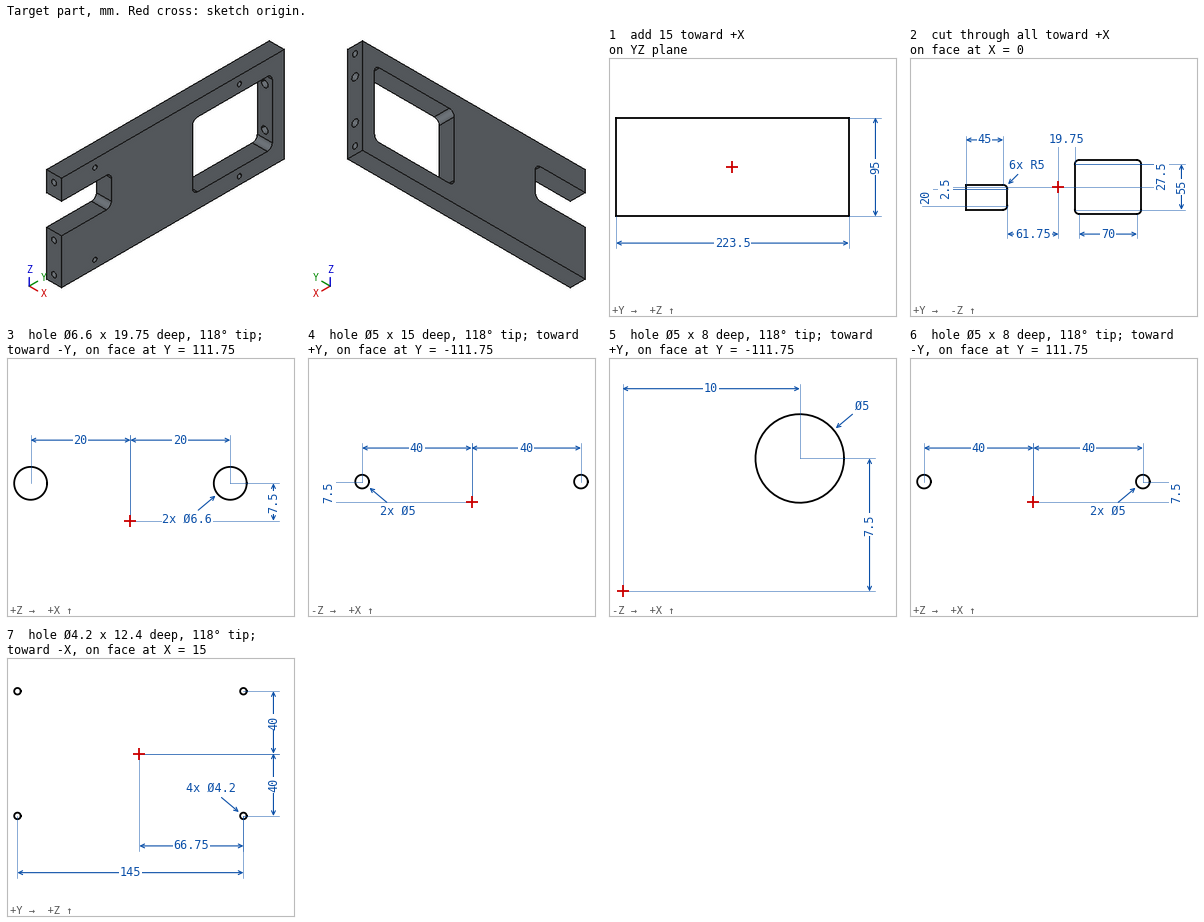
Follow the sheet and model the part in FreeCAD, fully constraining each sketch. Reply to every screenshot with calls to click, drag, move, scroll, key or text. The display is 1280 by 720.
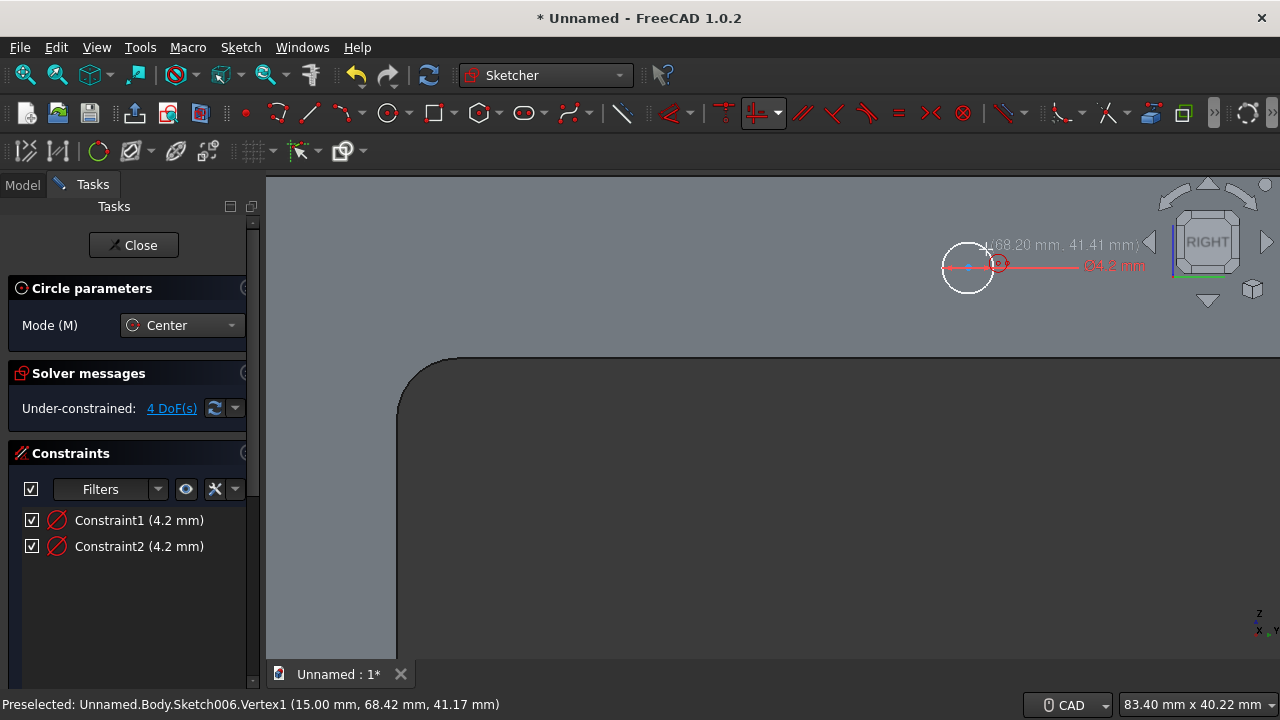
scroll(971, 268, down, 6)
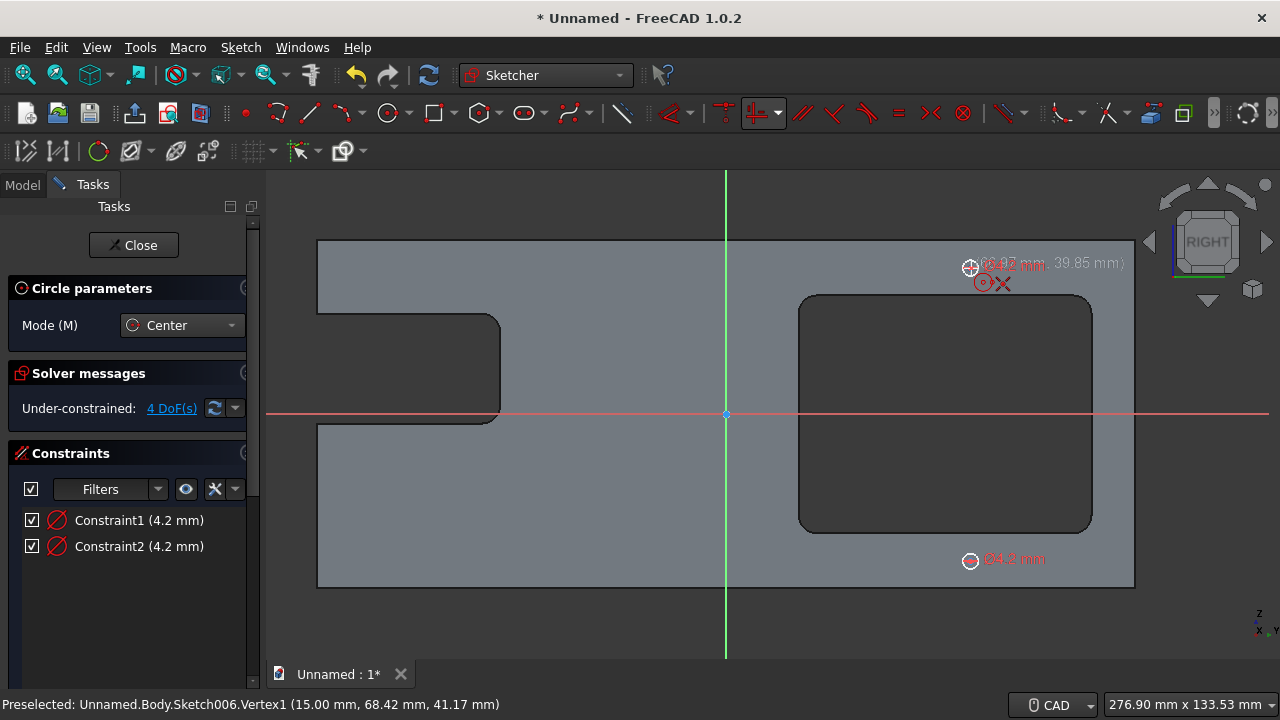
scroll(440, 561, up, 6)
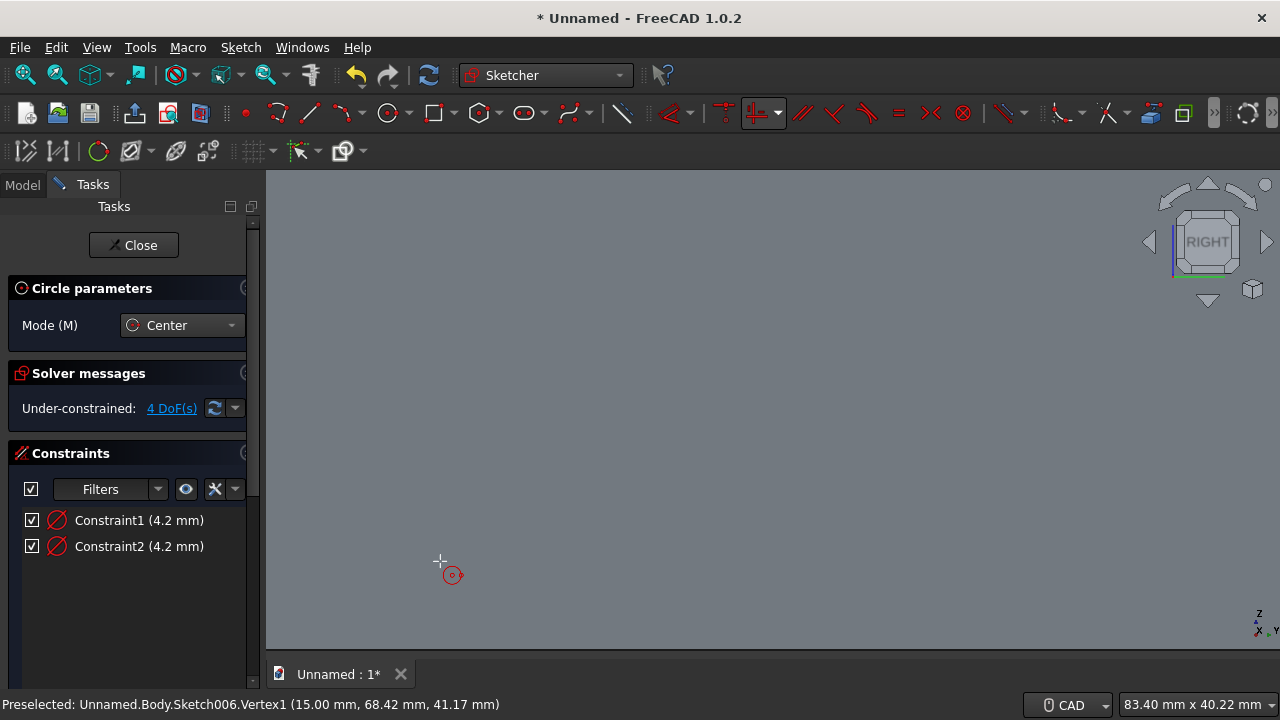
click(439, 559)
move(457, 541)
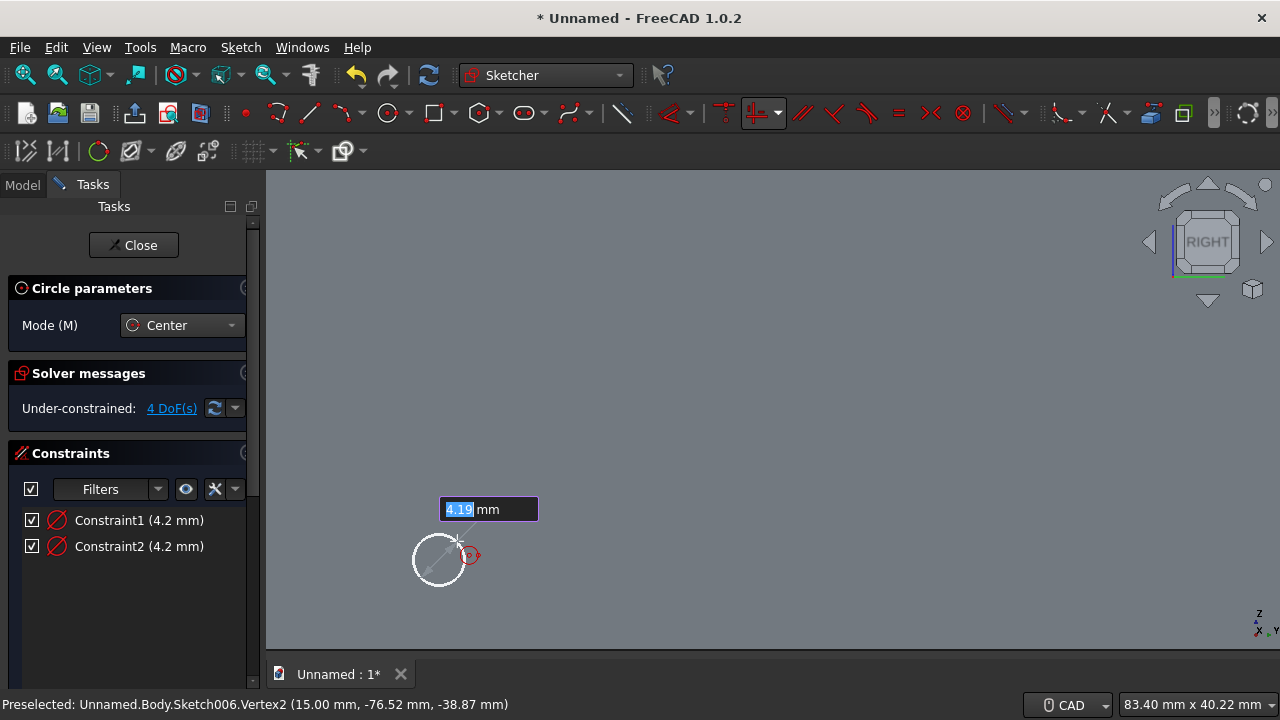
text(4.2)
key(Return)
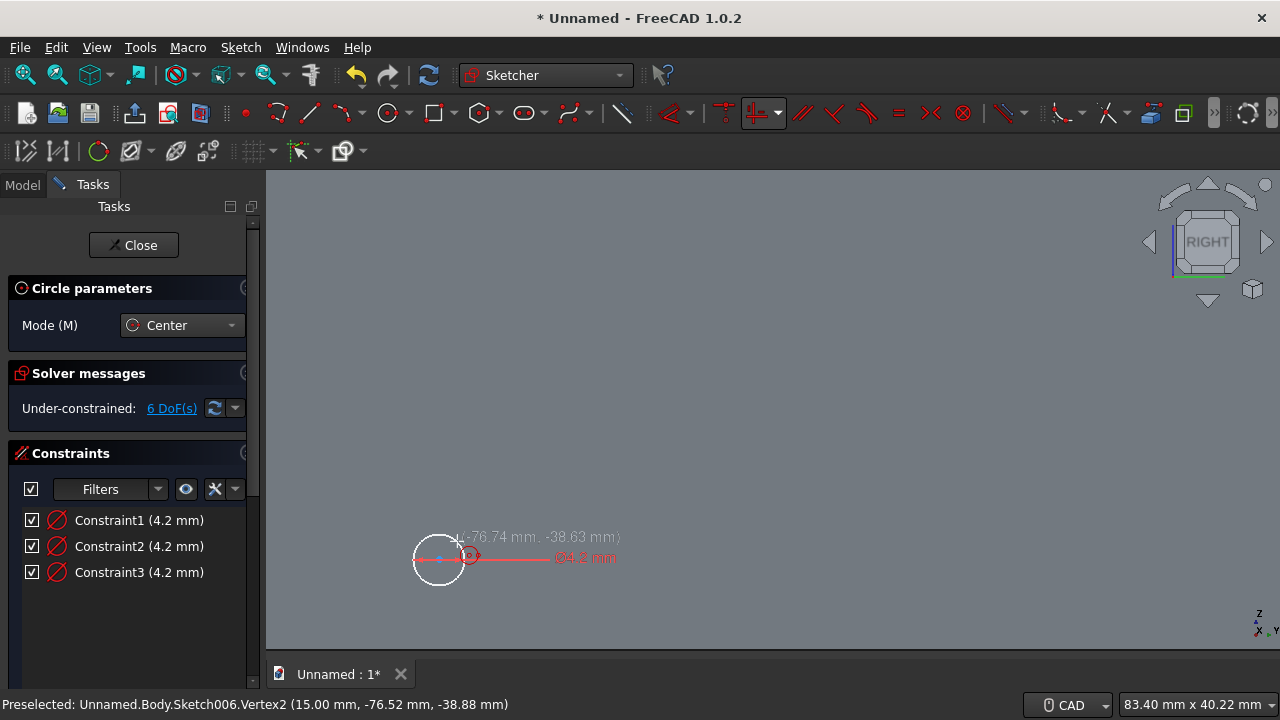
scroll(439, 562, down, 6)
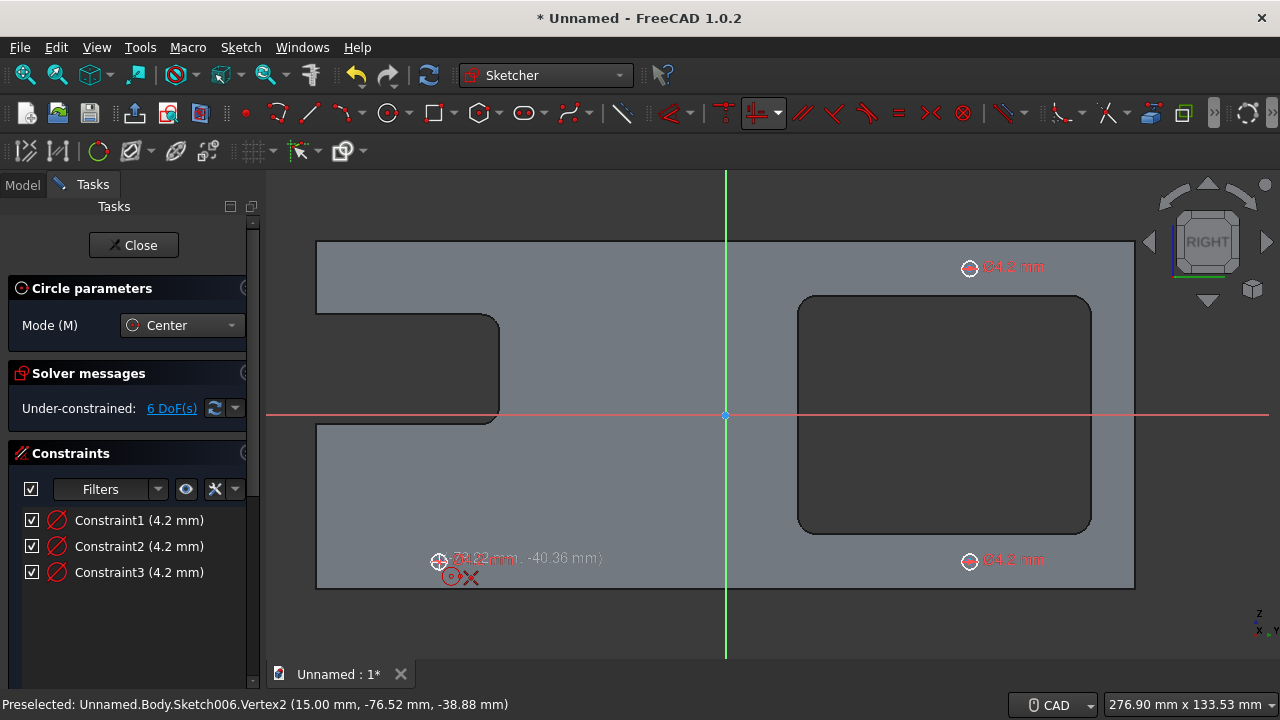
scroll(439, 269, up, 6)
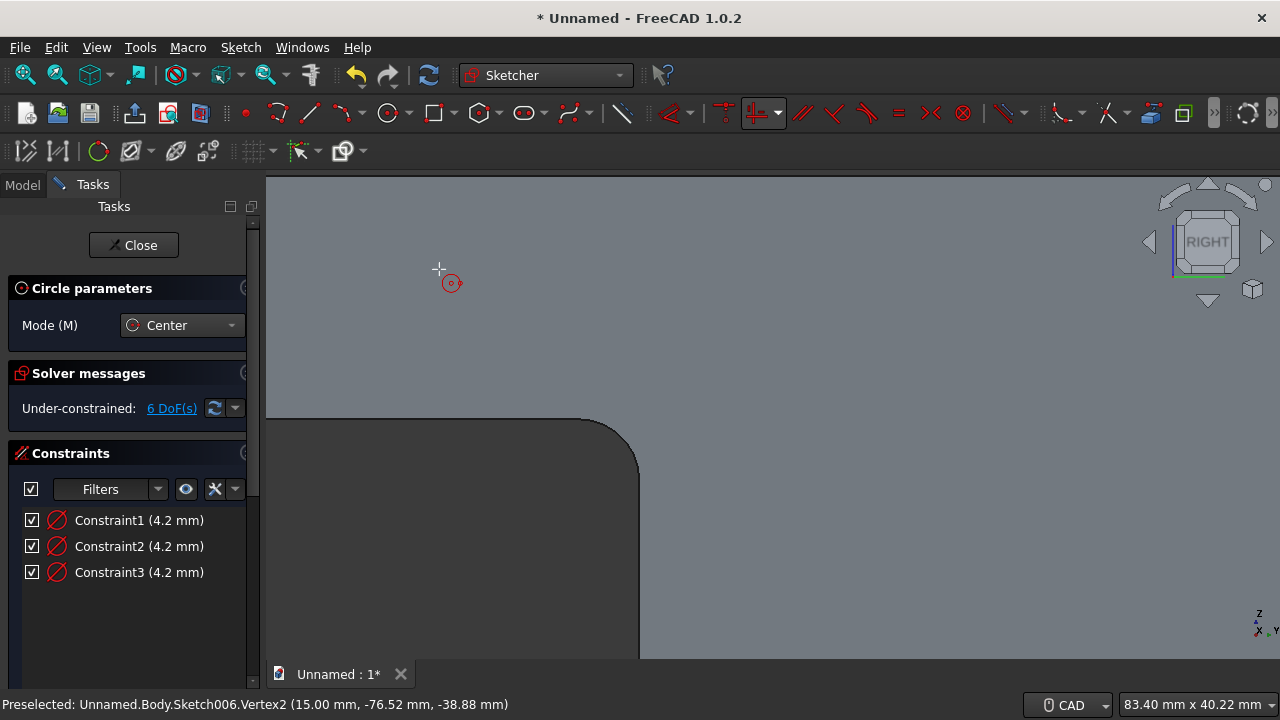
click(439, 267)
move(457, 249)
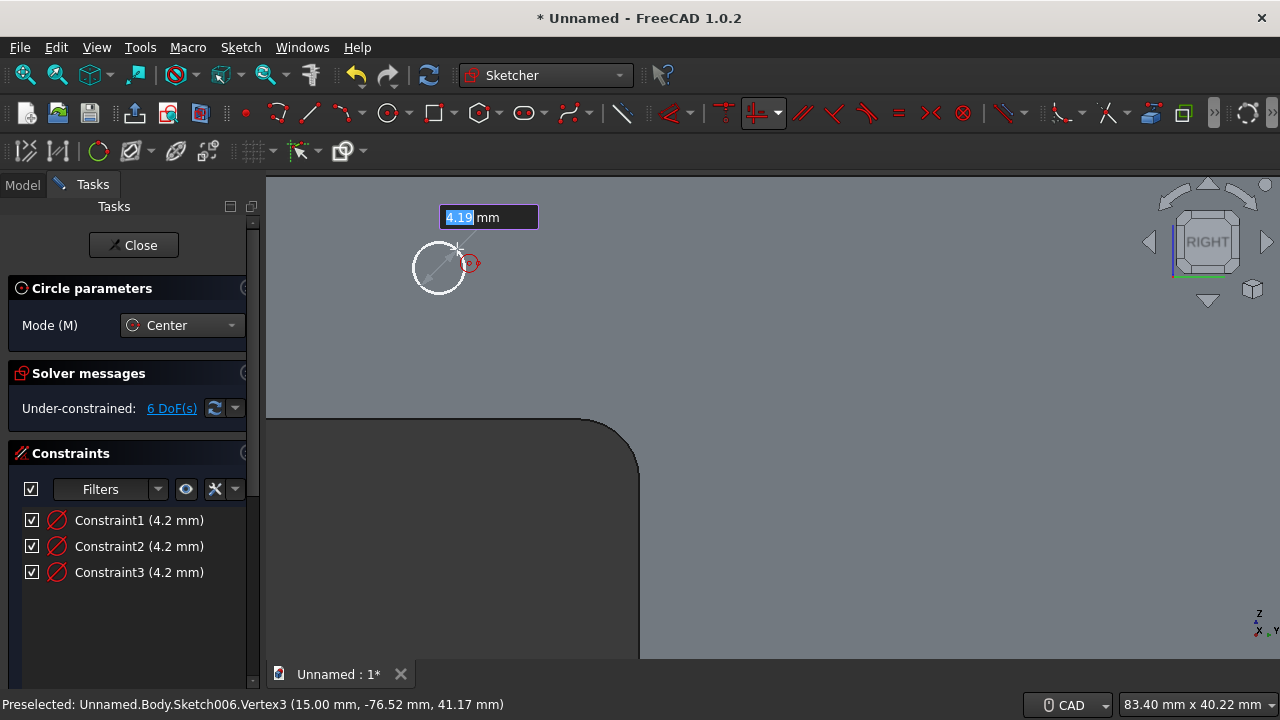
text(4.2)
key(Return)
key(Escape)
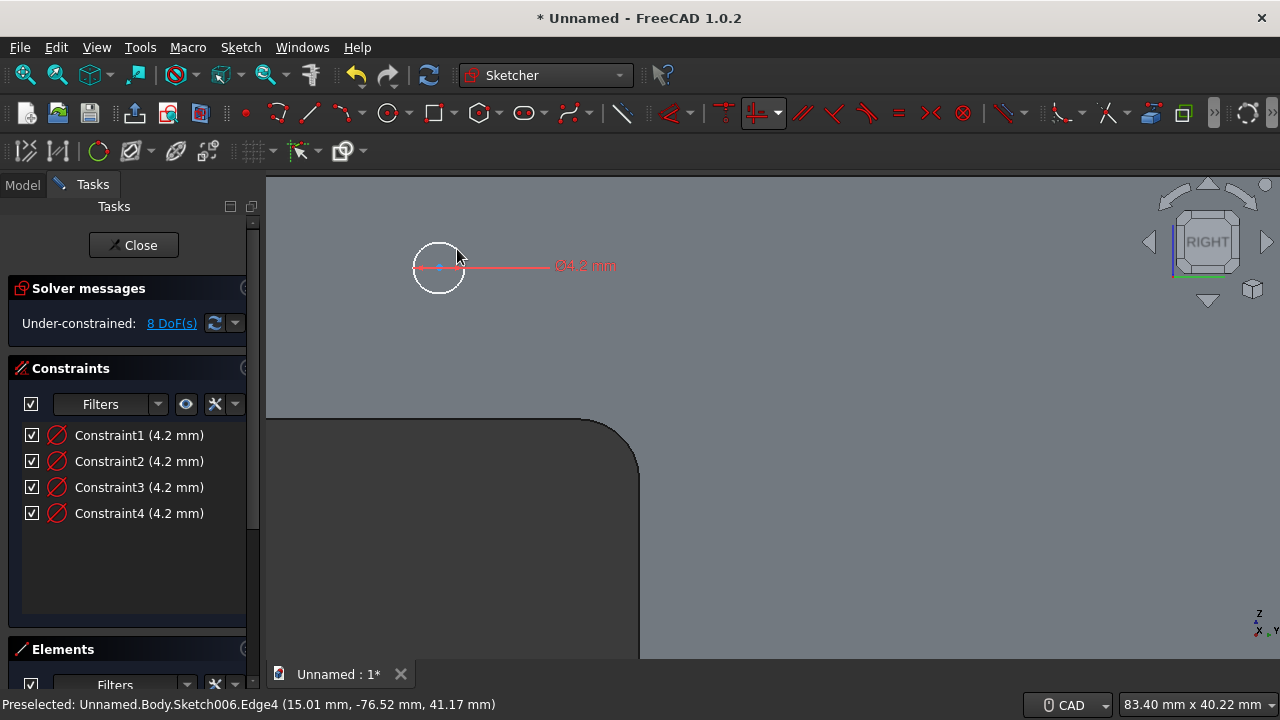
scroll(439, 268, down, 6)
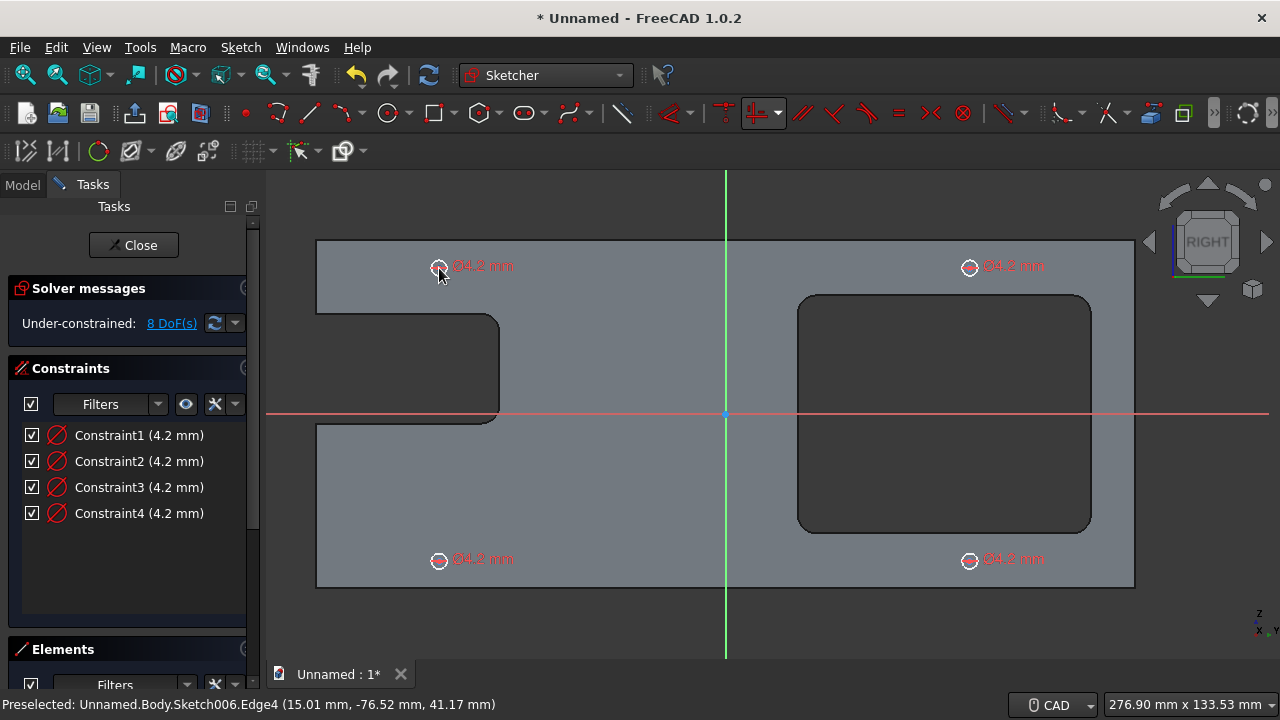
click(970, 561)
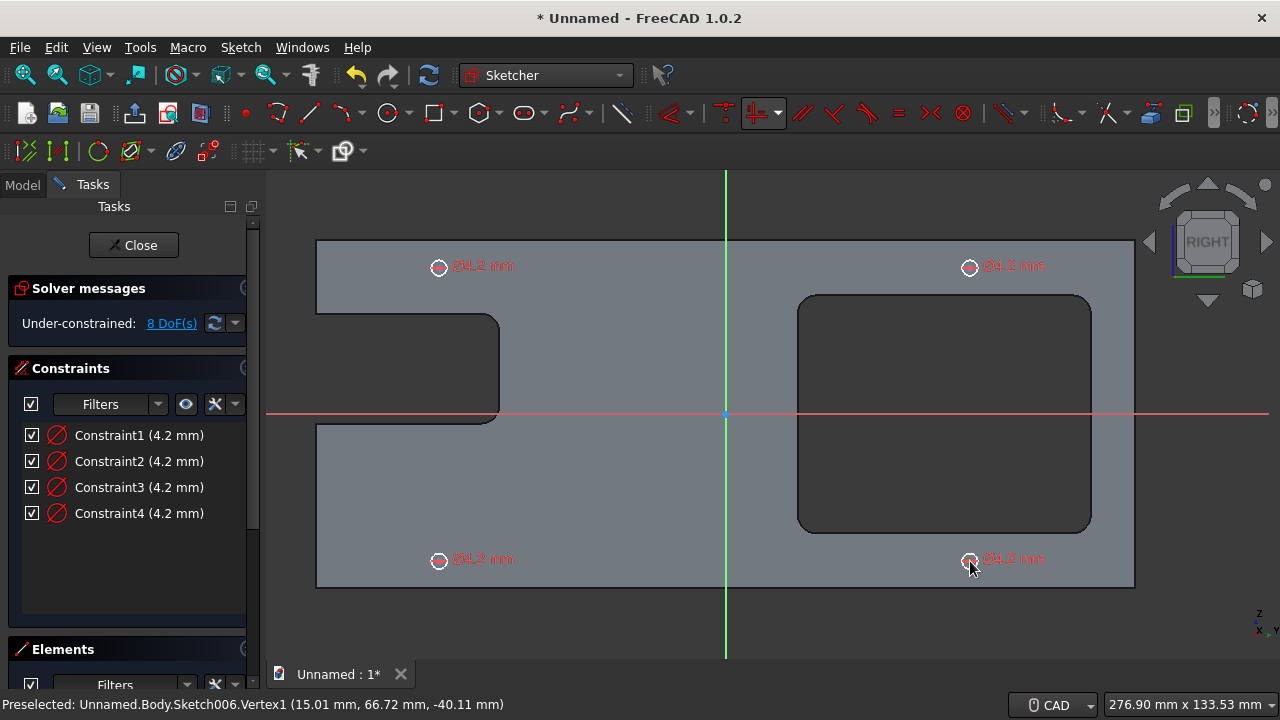
click(970, 268)